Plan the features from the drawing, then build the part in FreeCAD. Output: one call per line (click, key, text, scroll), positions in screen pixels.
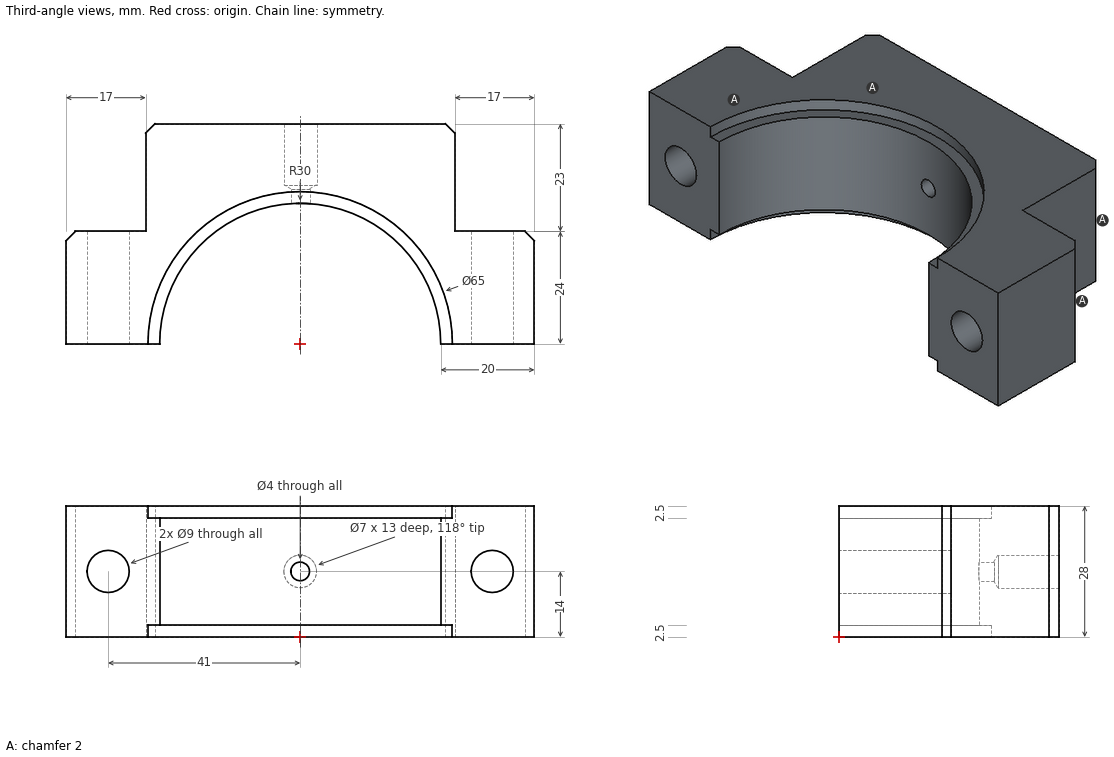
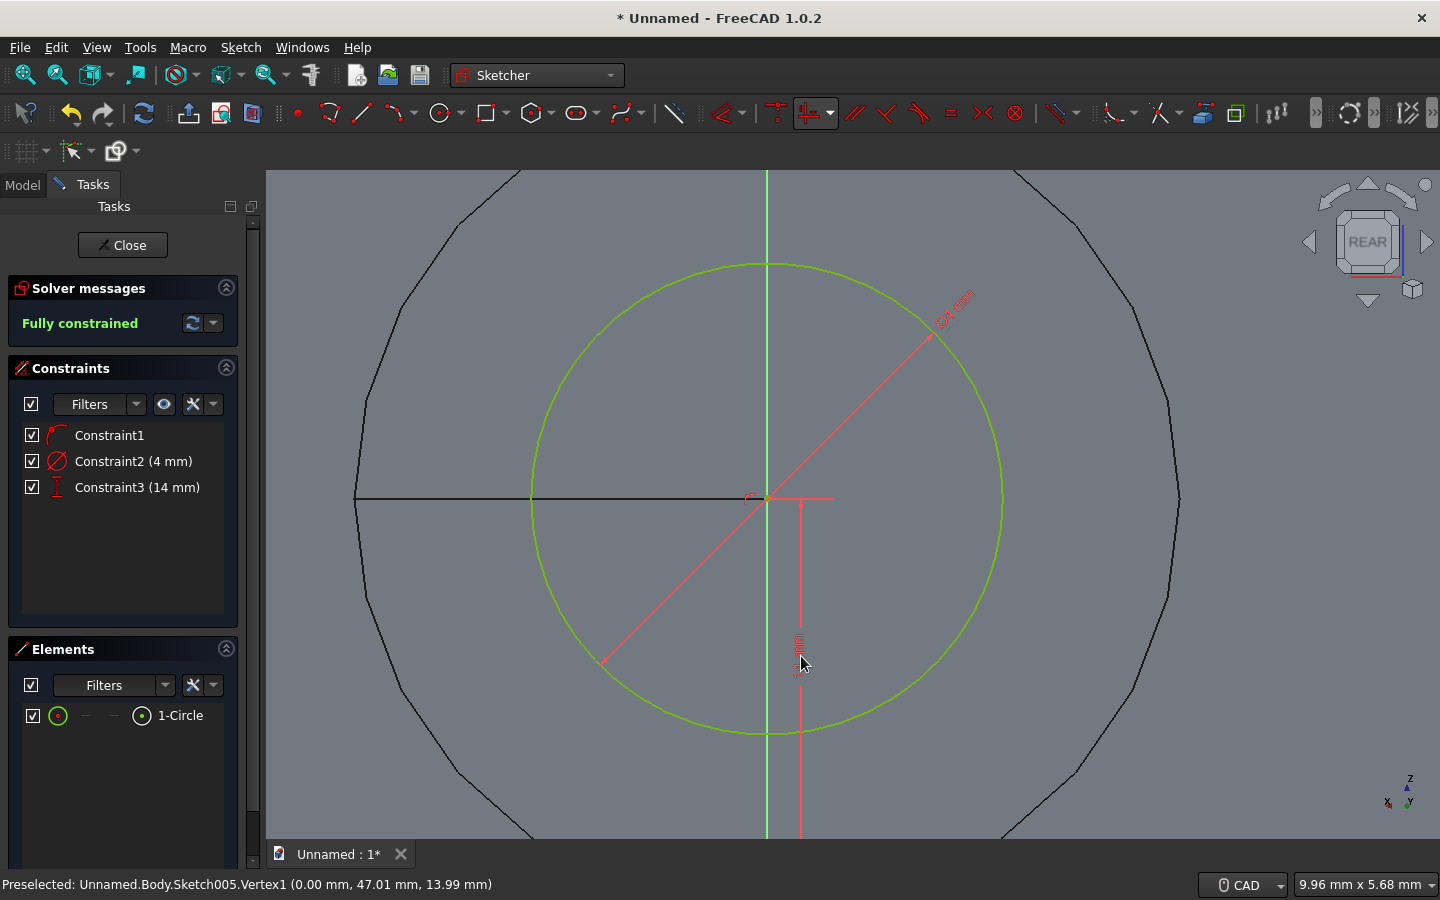
click(123, 245)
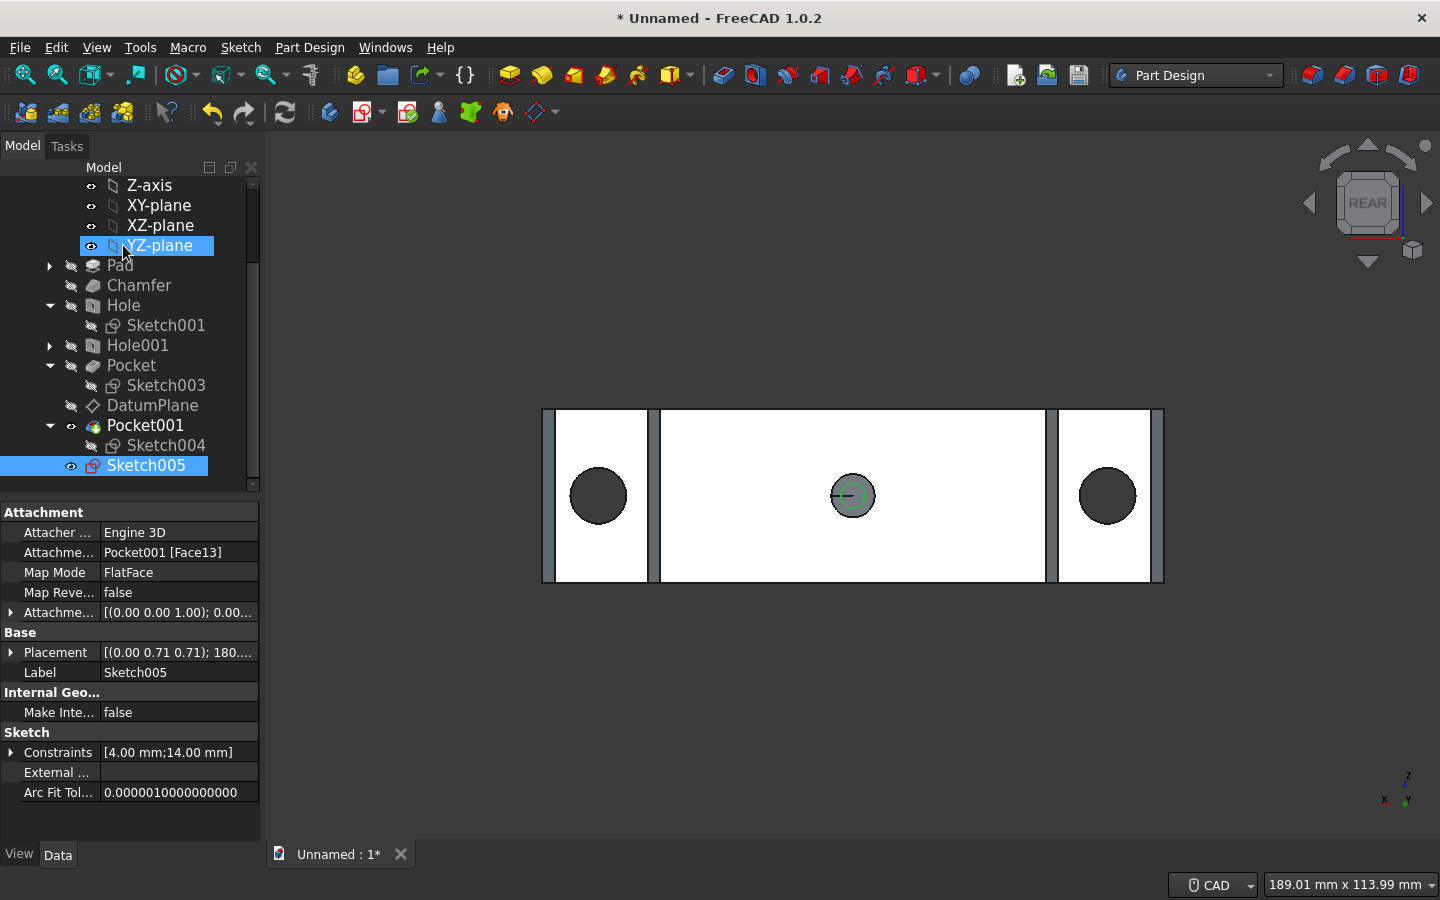
click(756, 76)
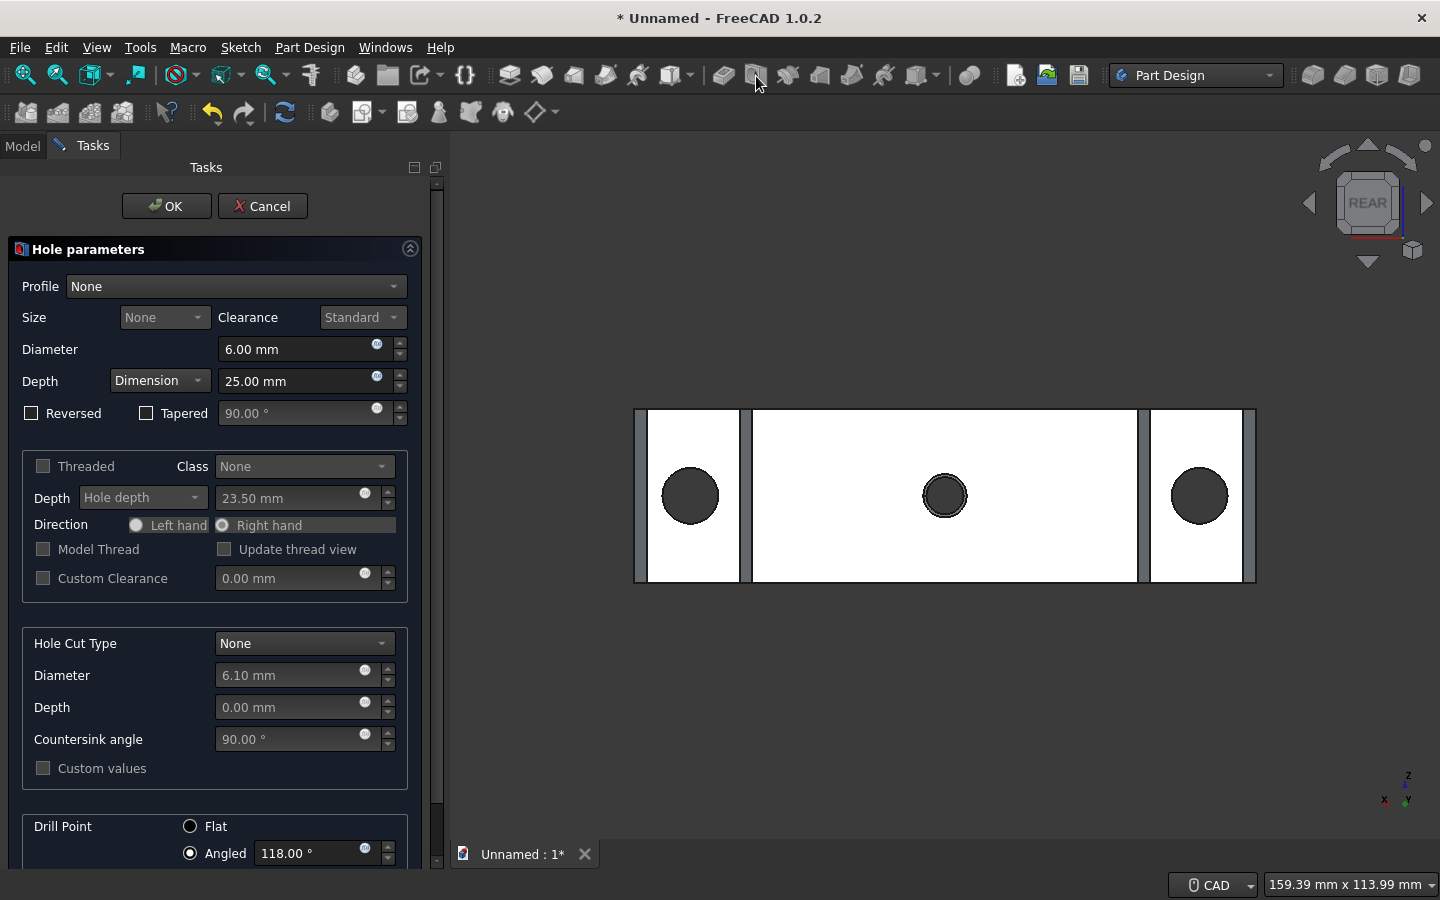
triple_click(305, 349)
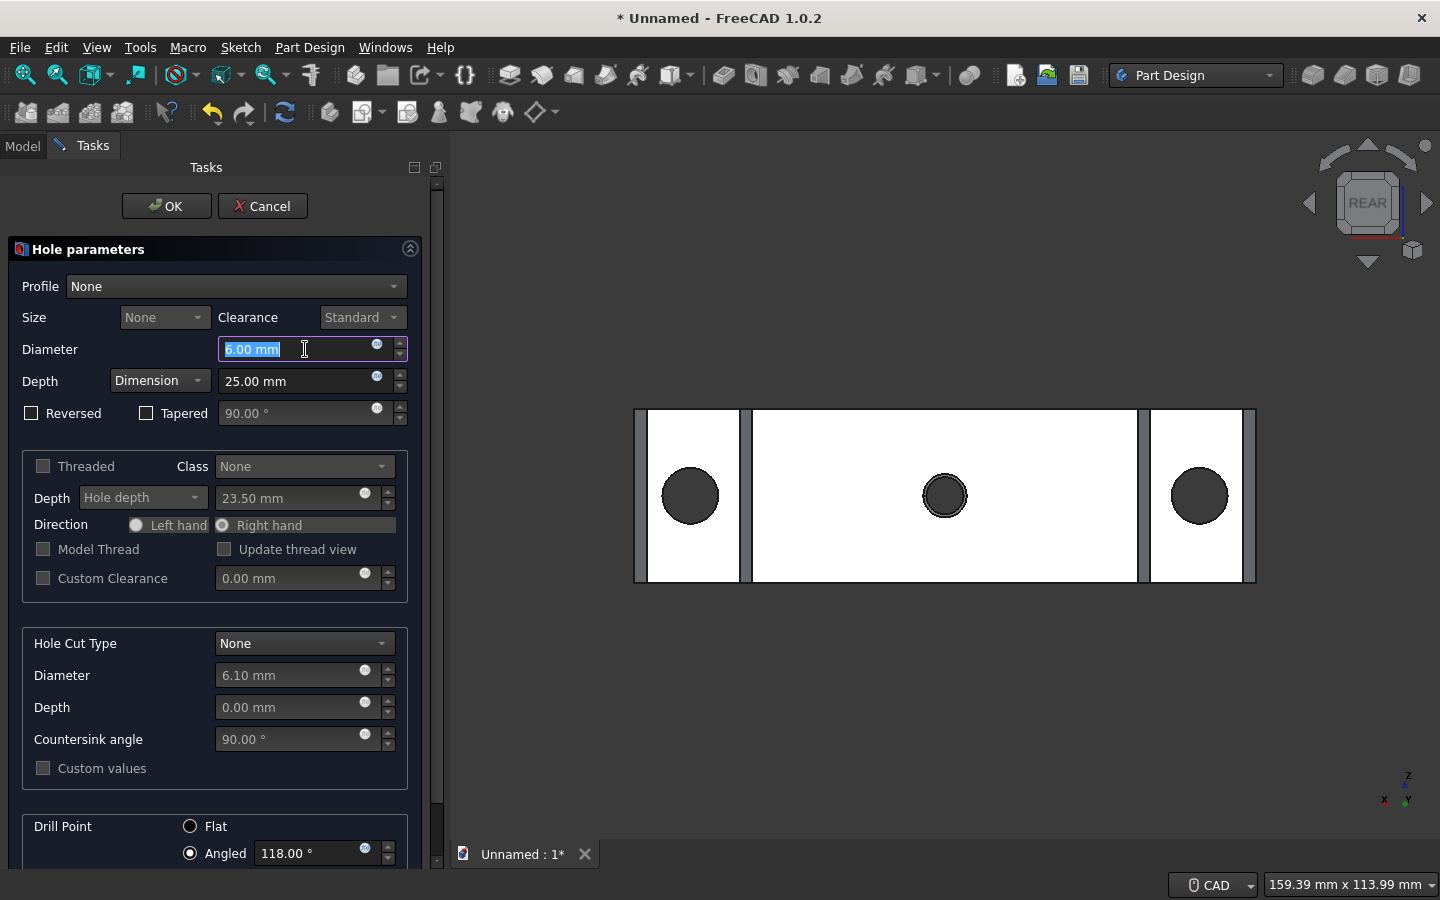
text(4)
key(Tab)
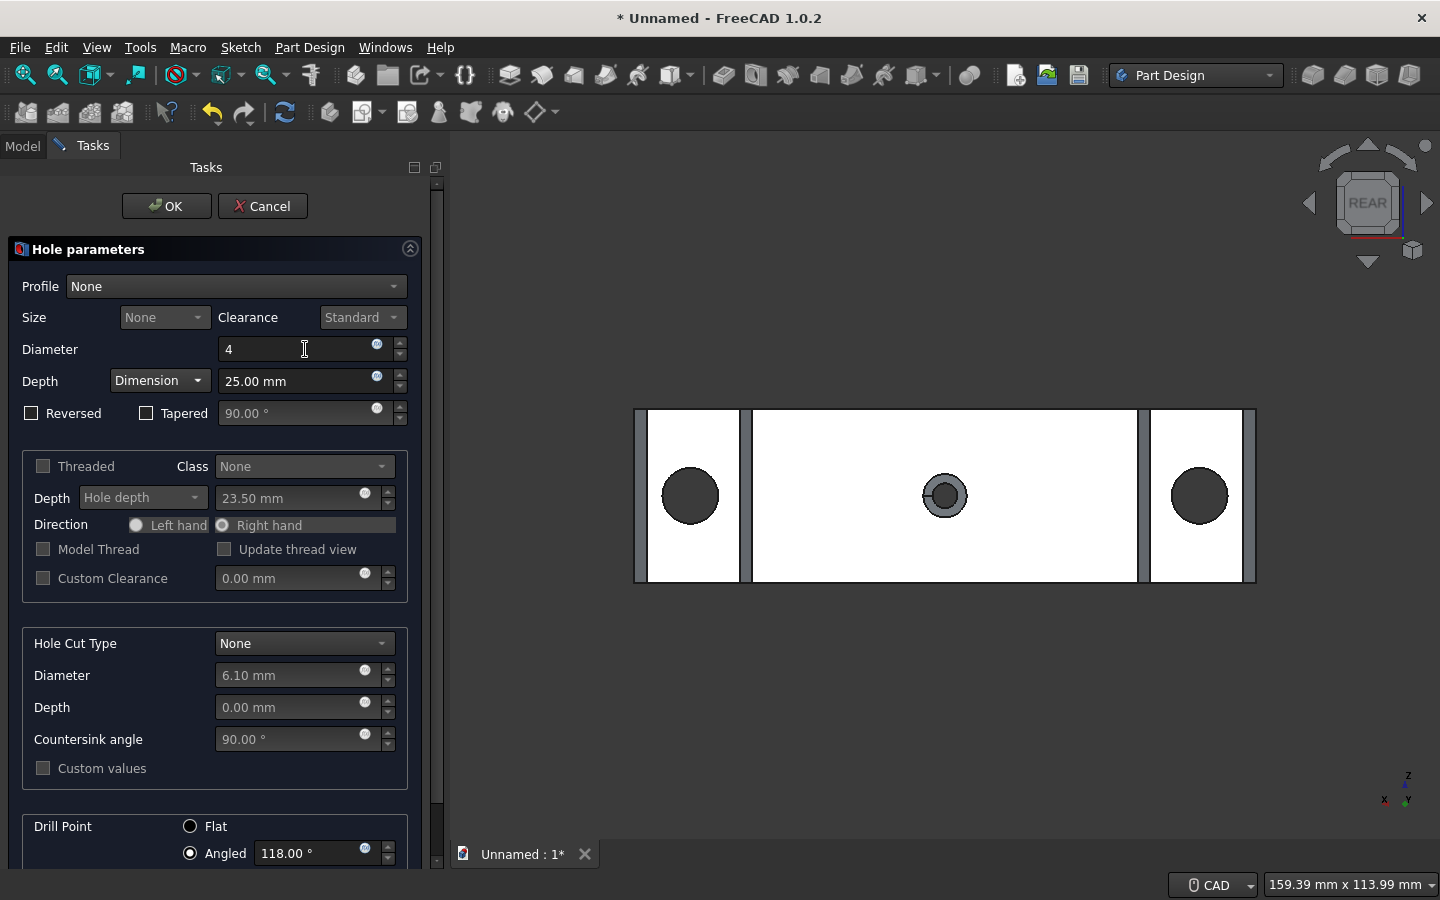
click(161, 380)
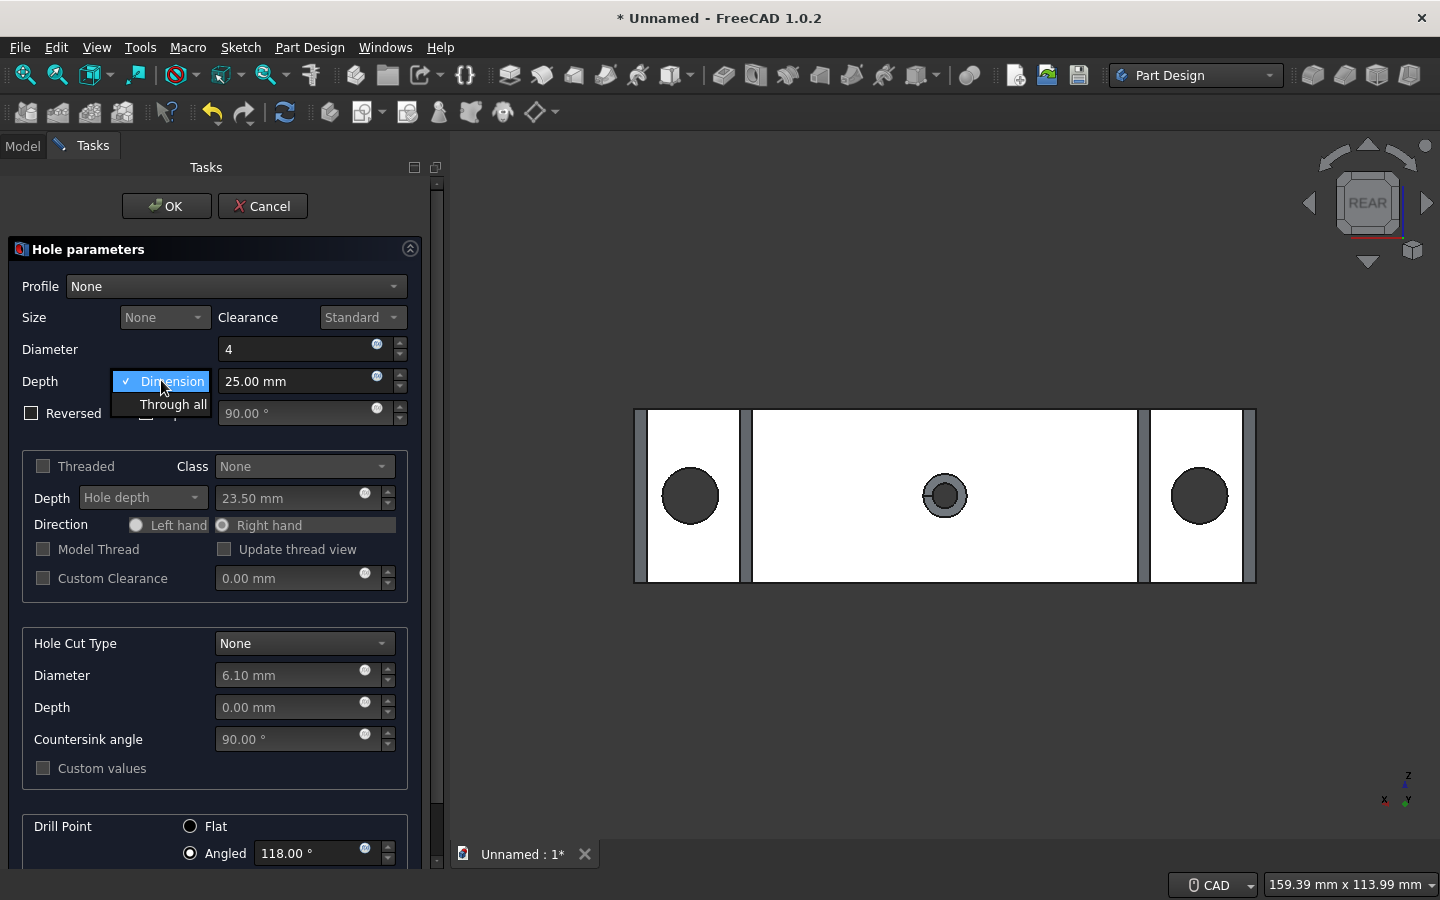
click(160, 404)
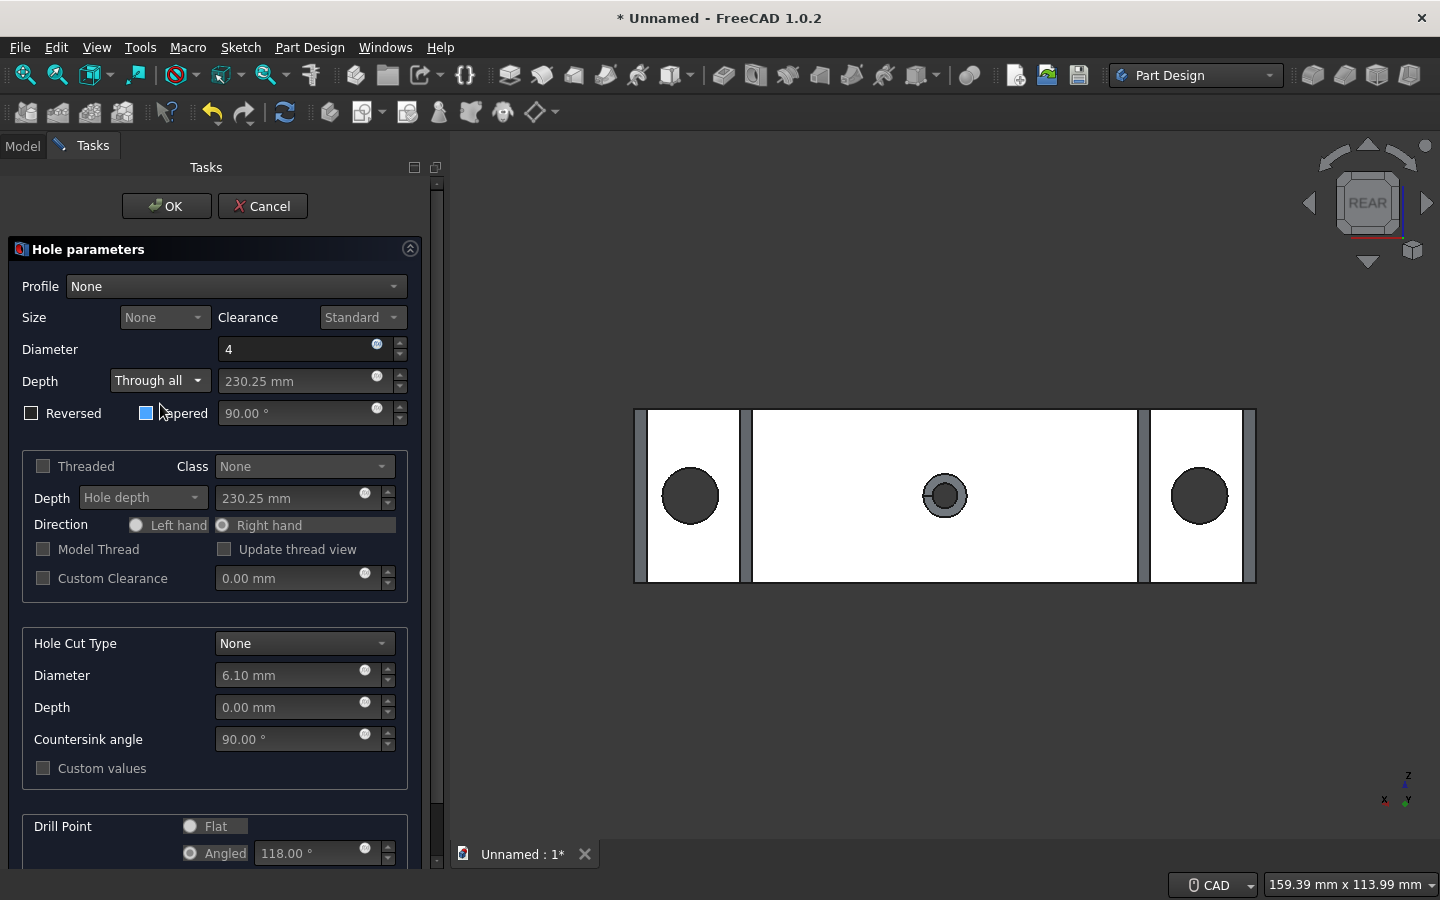
click(167, 206)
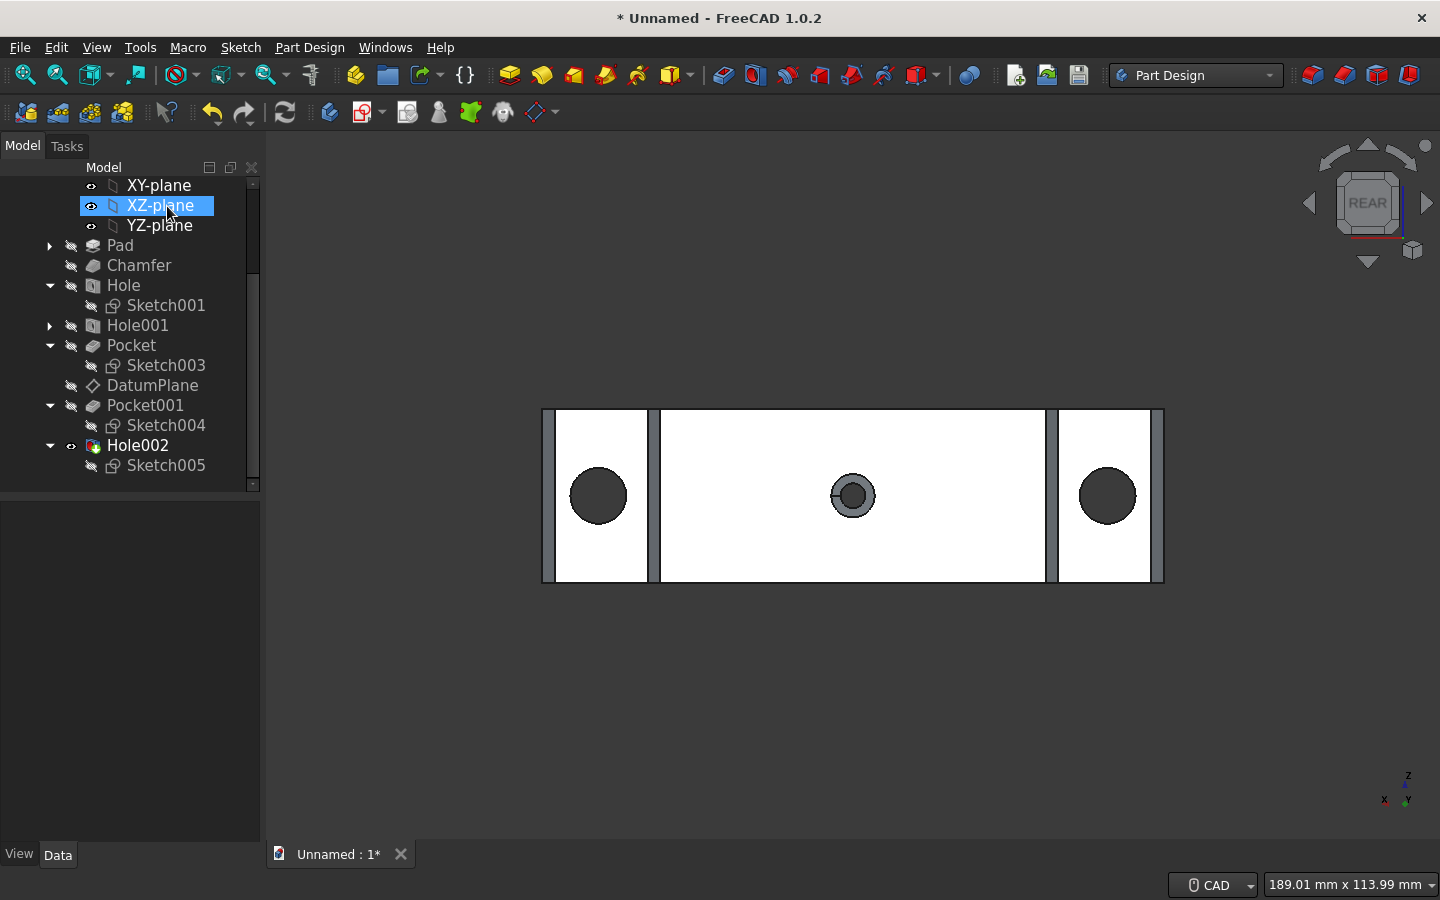
key(0)